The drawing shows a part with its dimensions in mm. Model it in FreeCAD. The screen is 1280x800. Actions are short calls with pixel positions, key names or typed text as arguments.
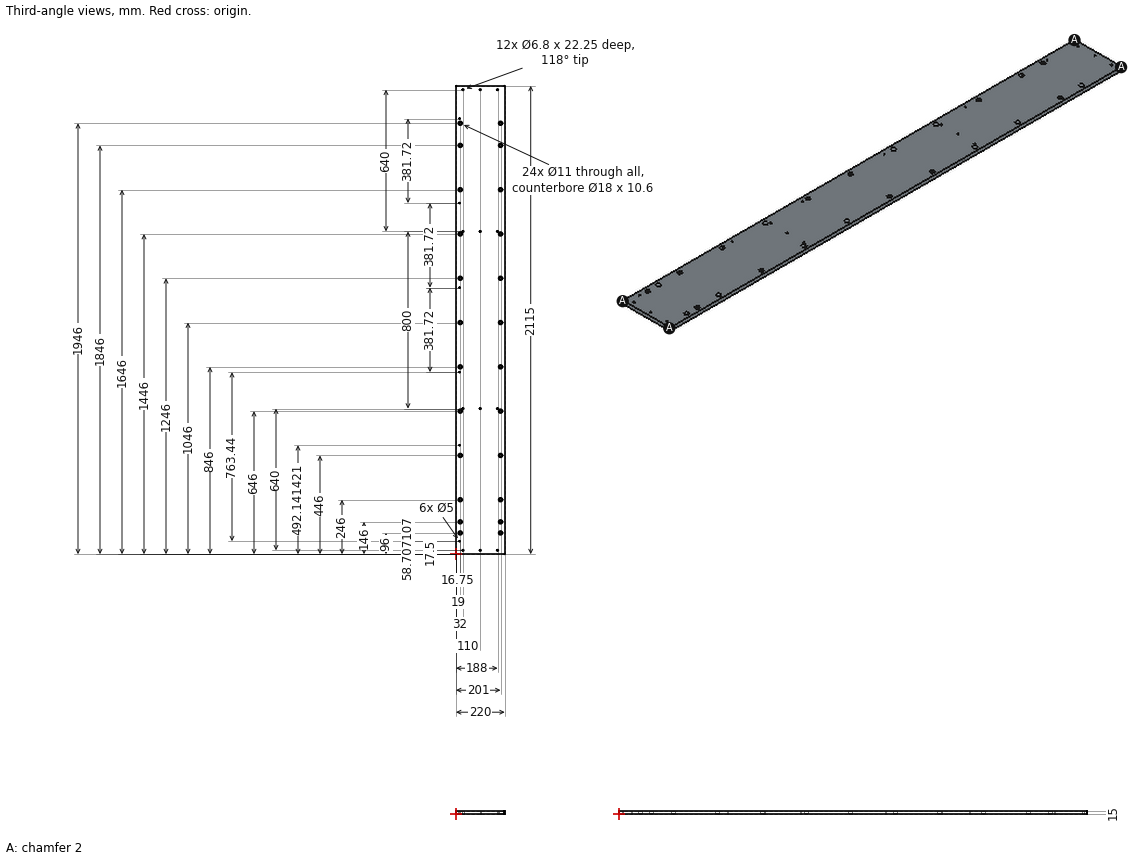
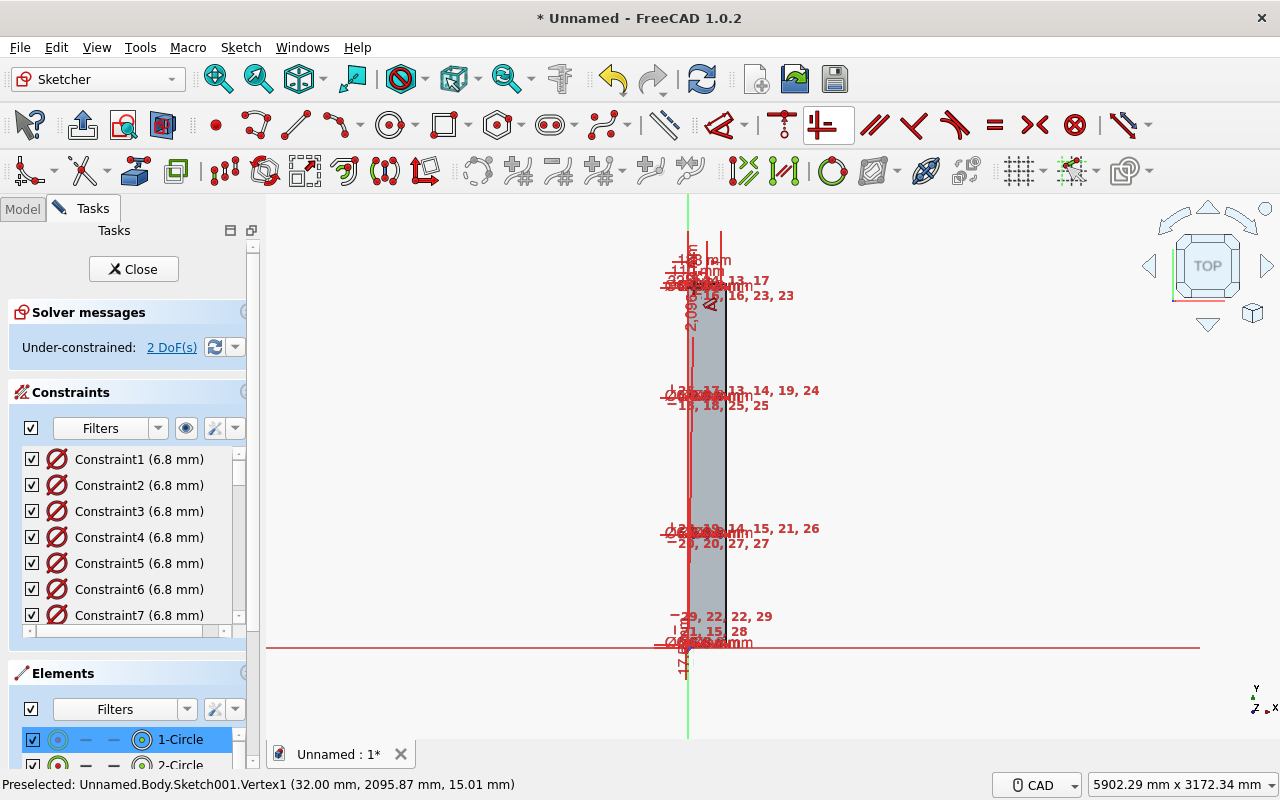
click(694, 398)
click(660, 343)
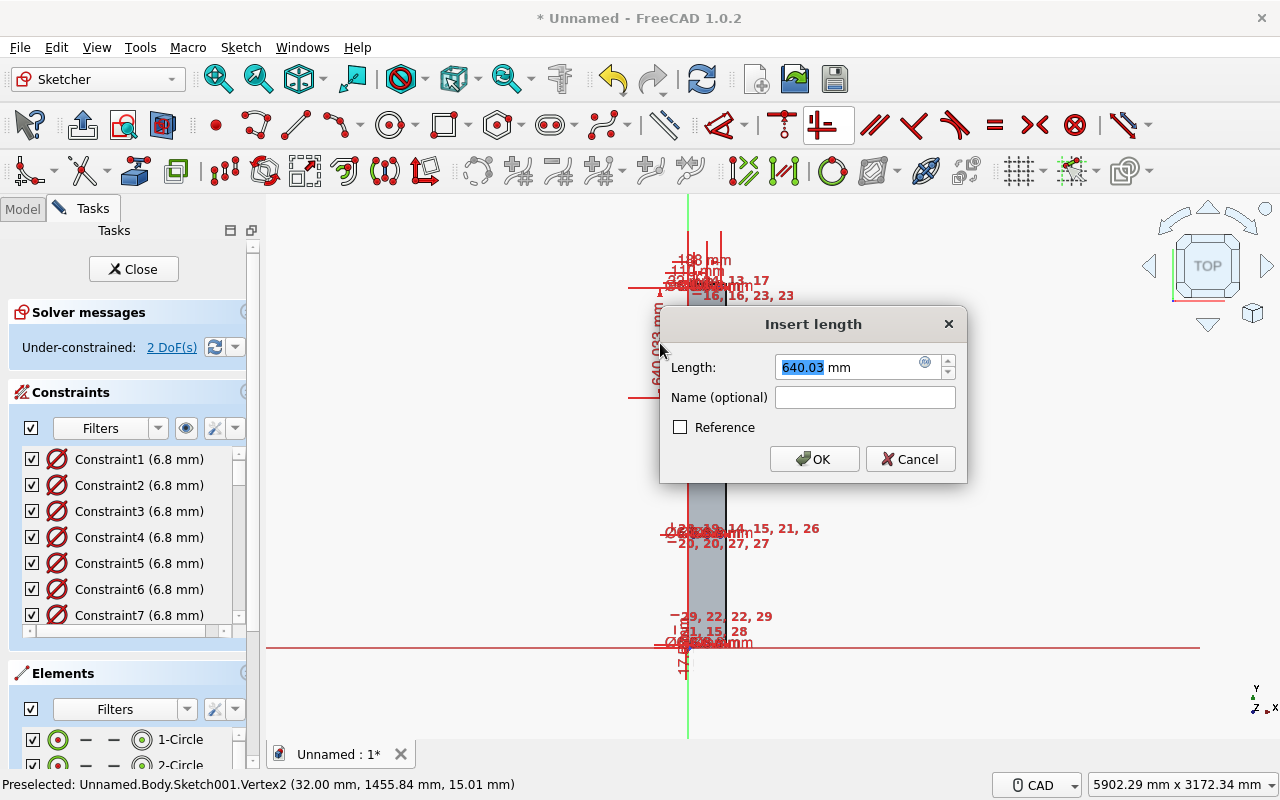
text(640)
key(Return)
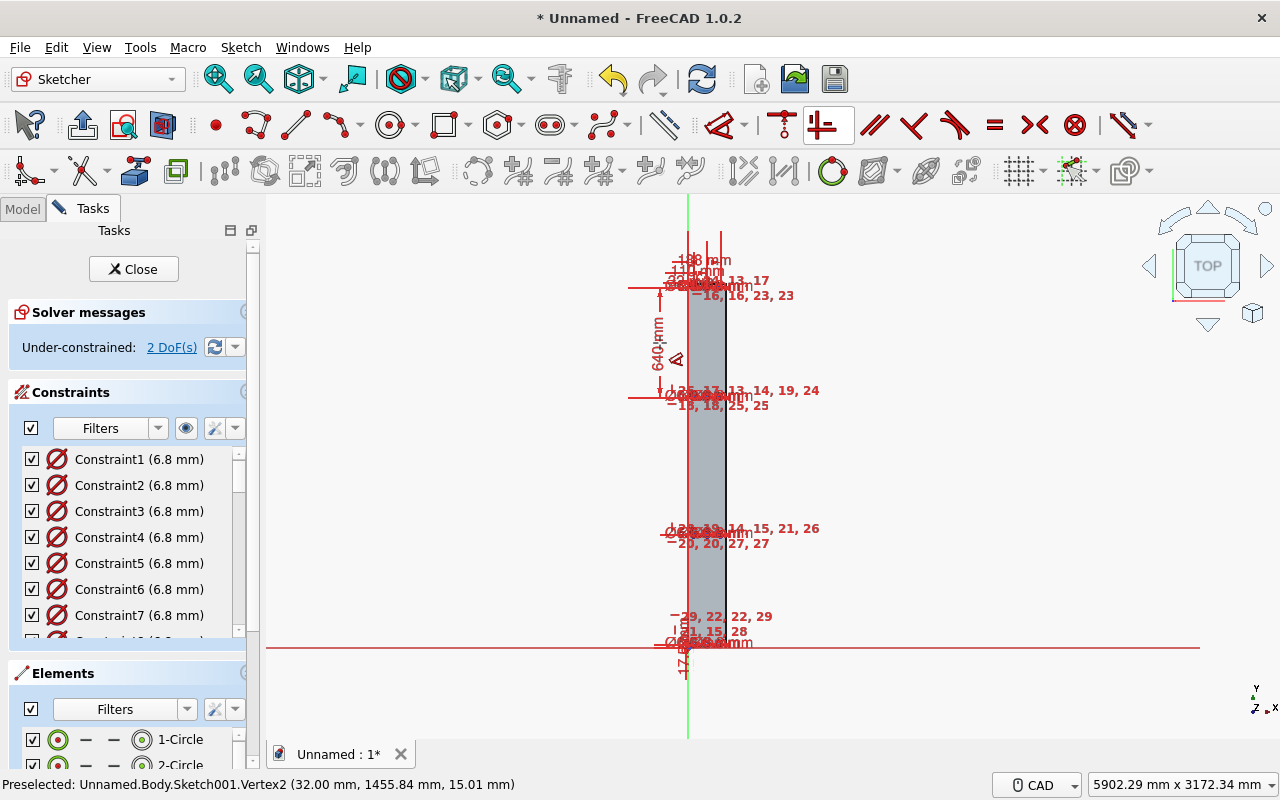
click(694, 398)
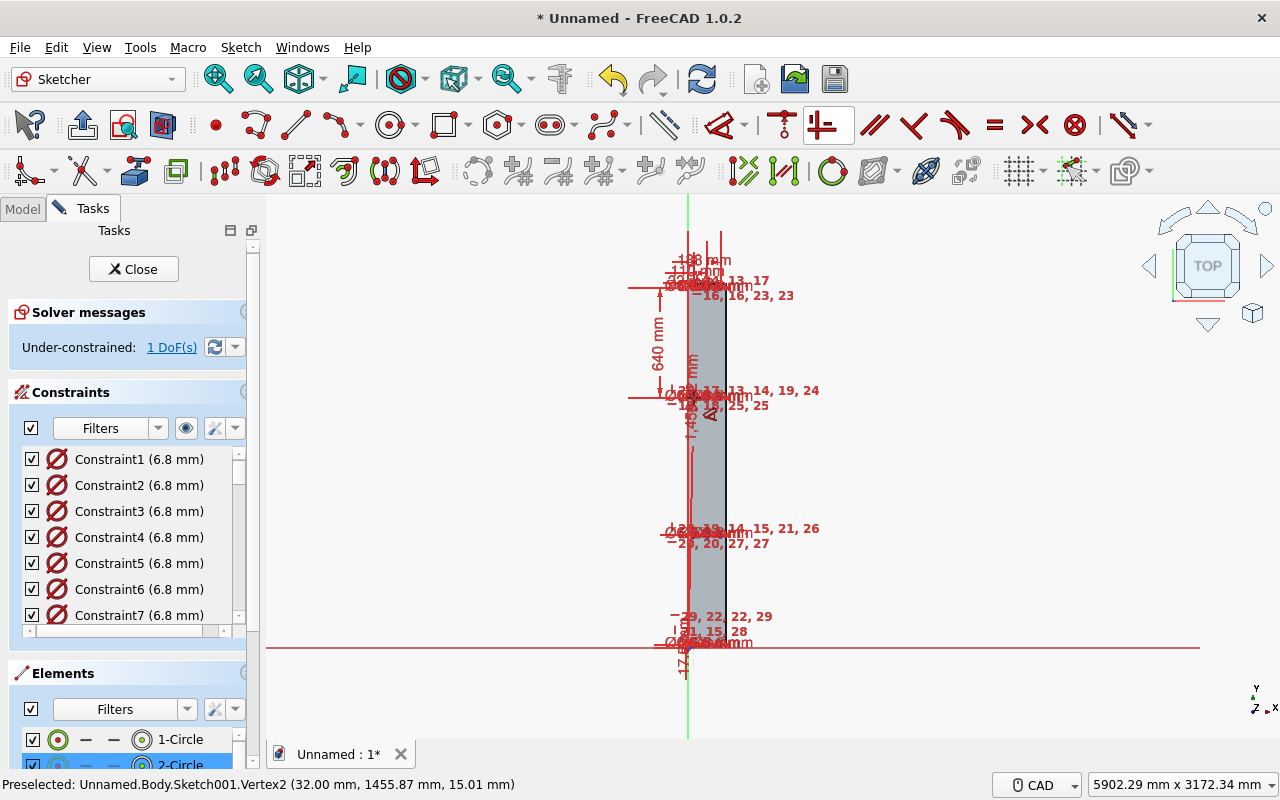
click(694, 535)
click(660, 466)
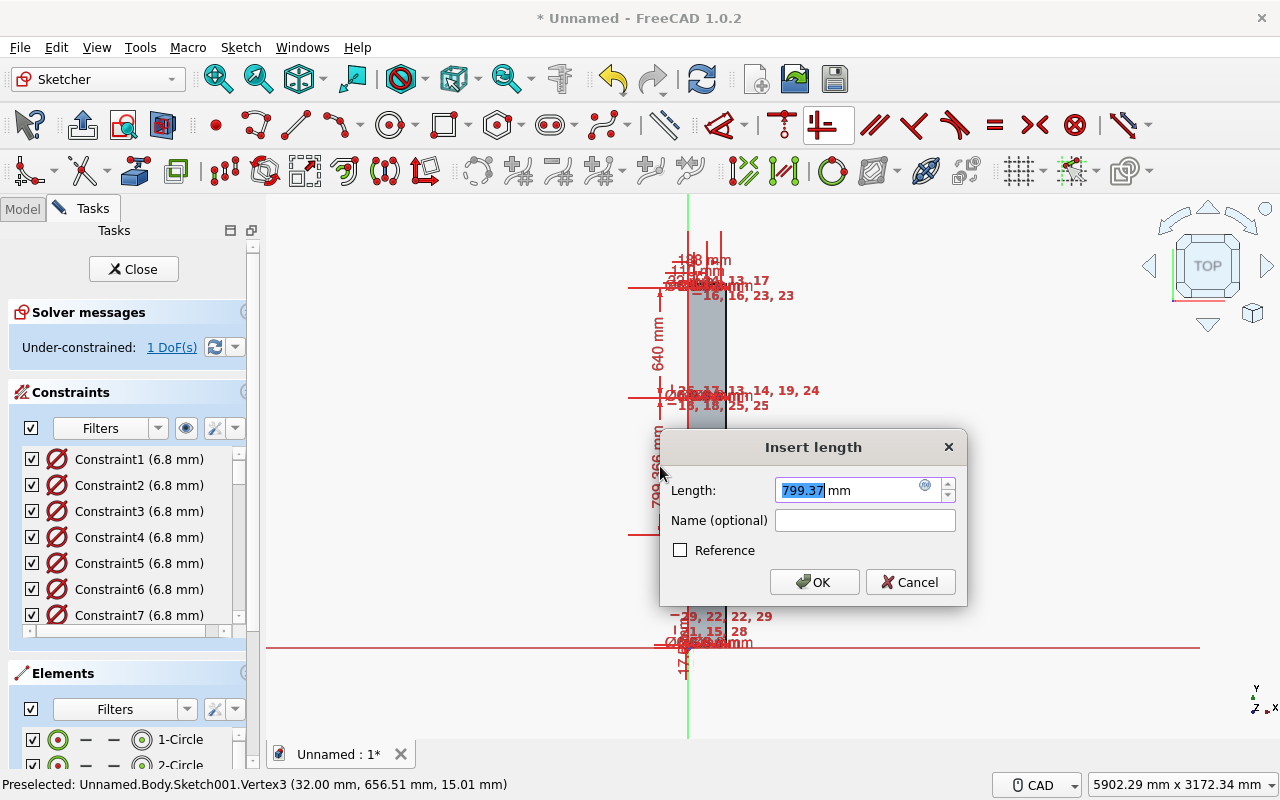
text(800)
key(Return)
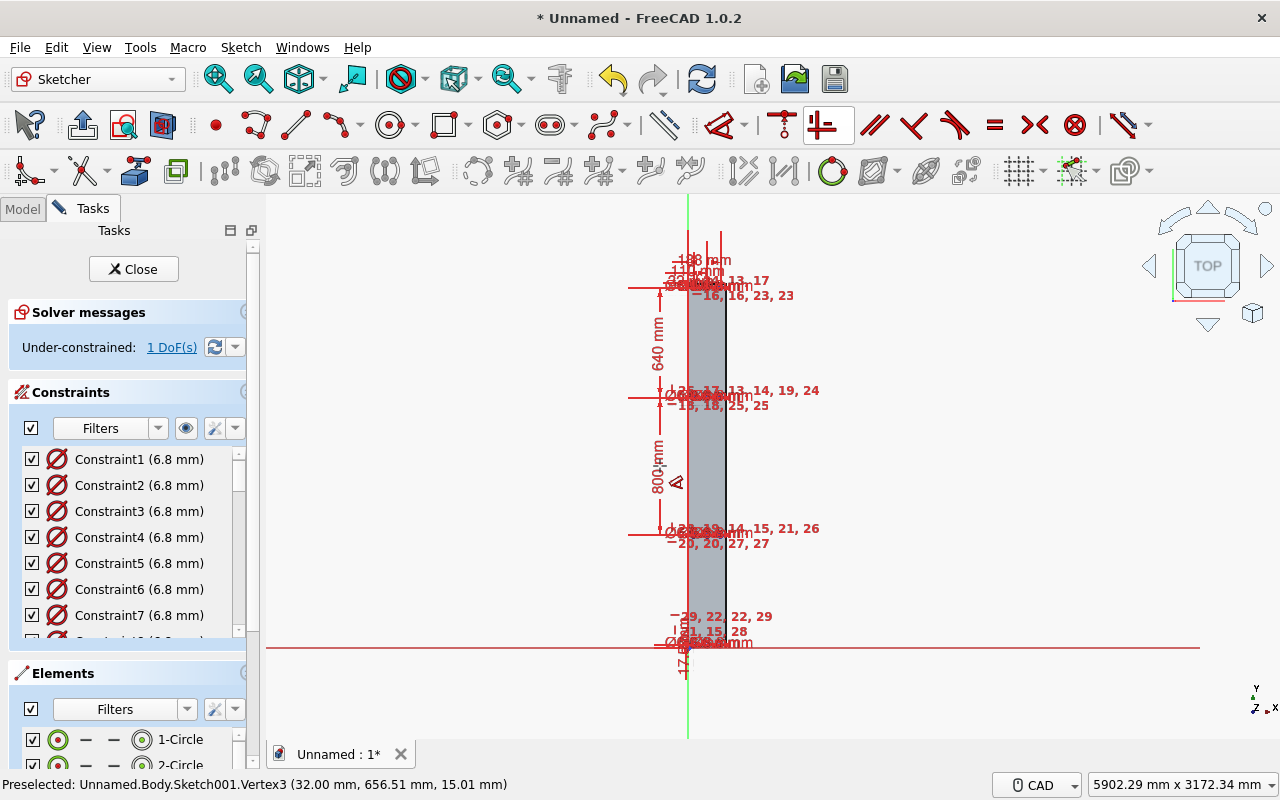
click(694, 535)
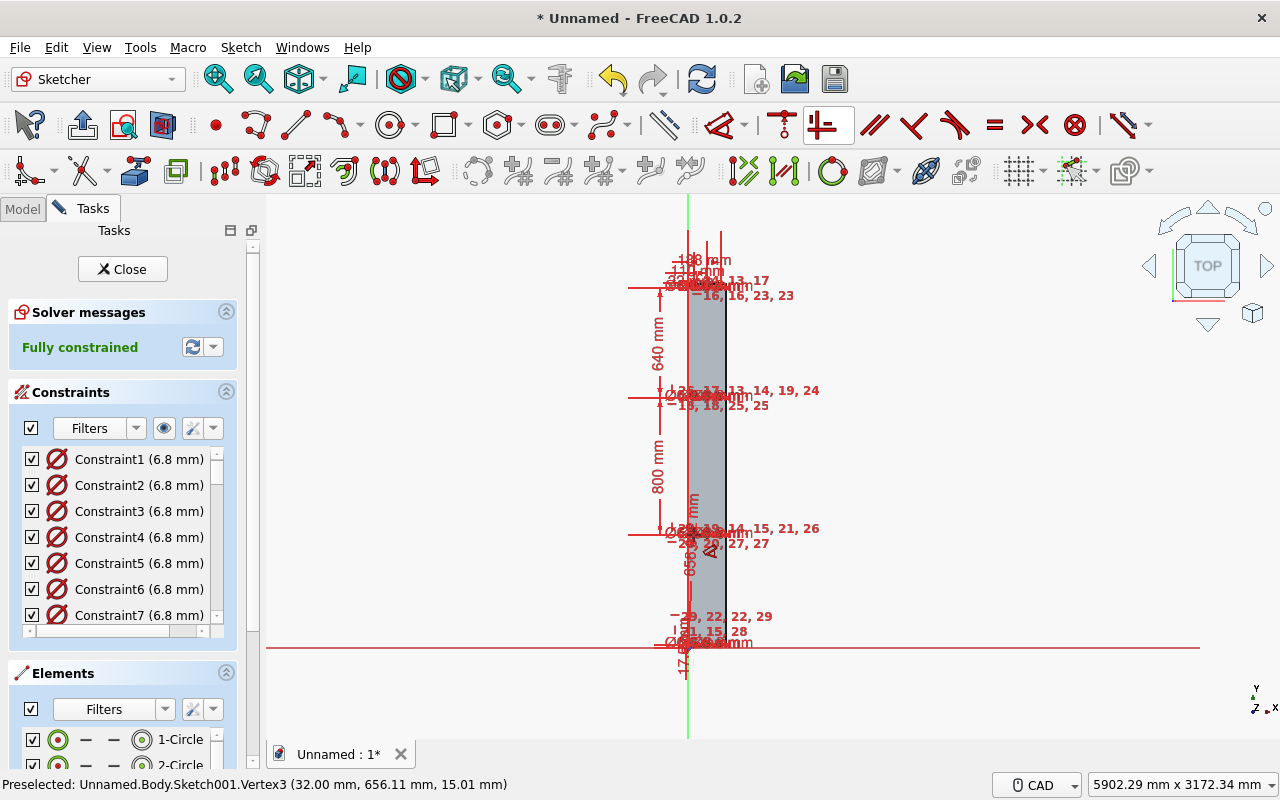
scroll(694, 645, up, 4)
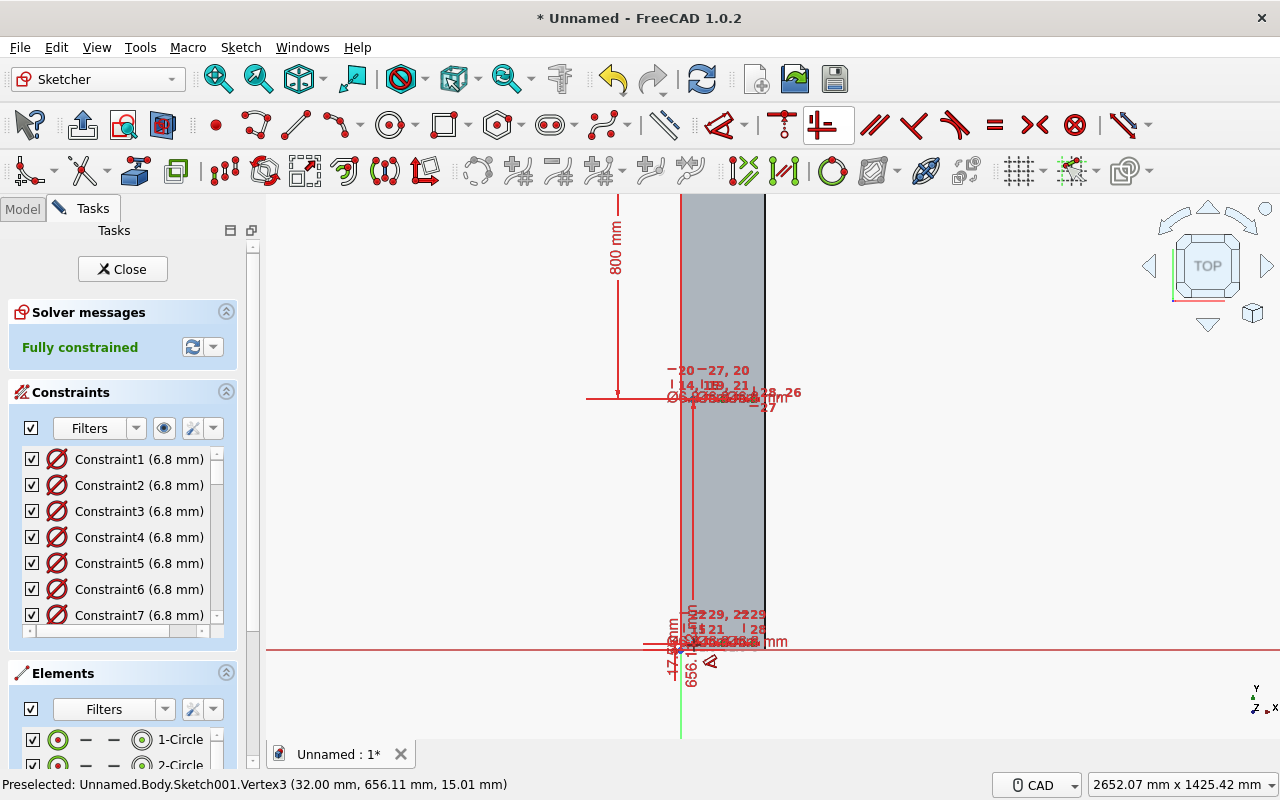
click(693, 644)
click(659, 522)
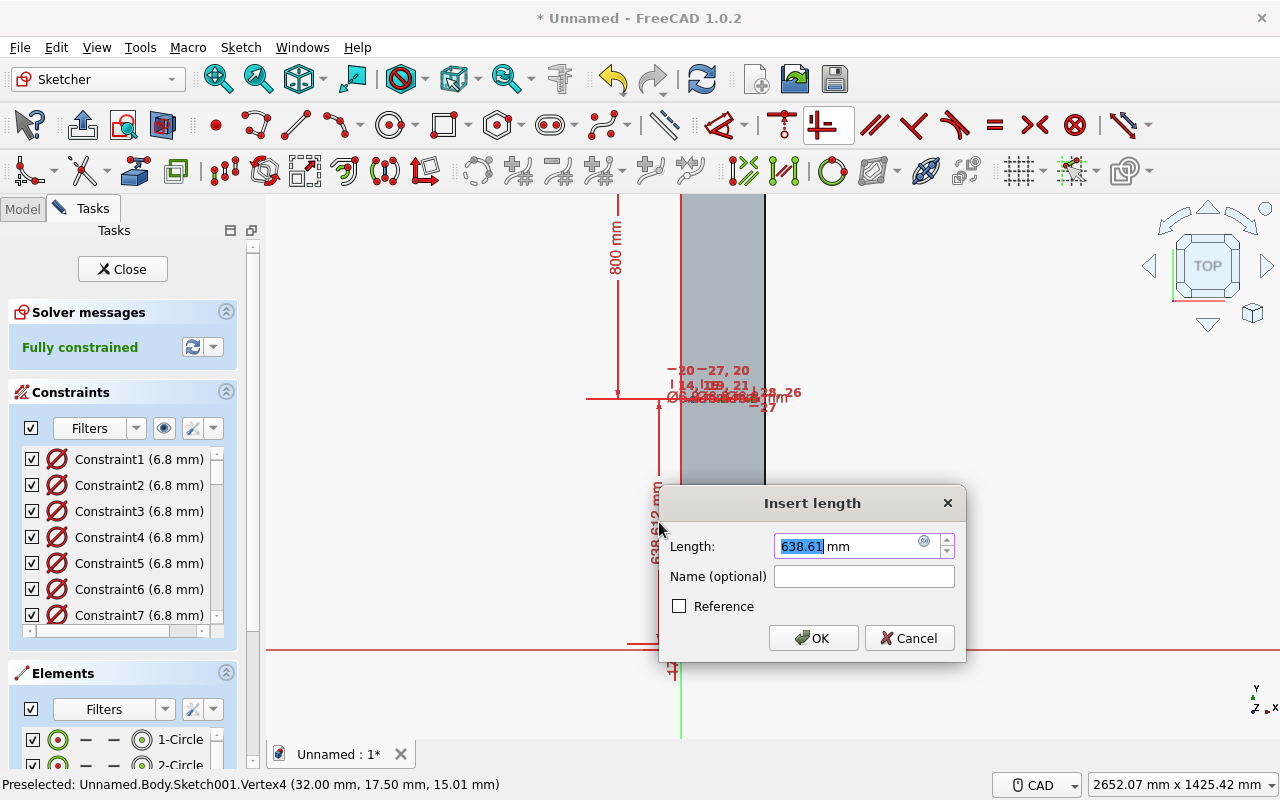
text(640)
key(Return)
key(Escape)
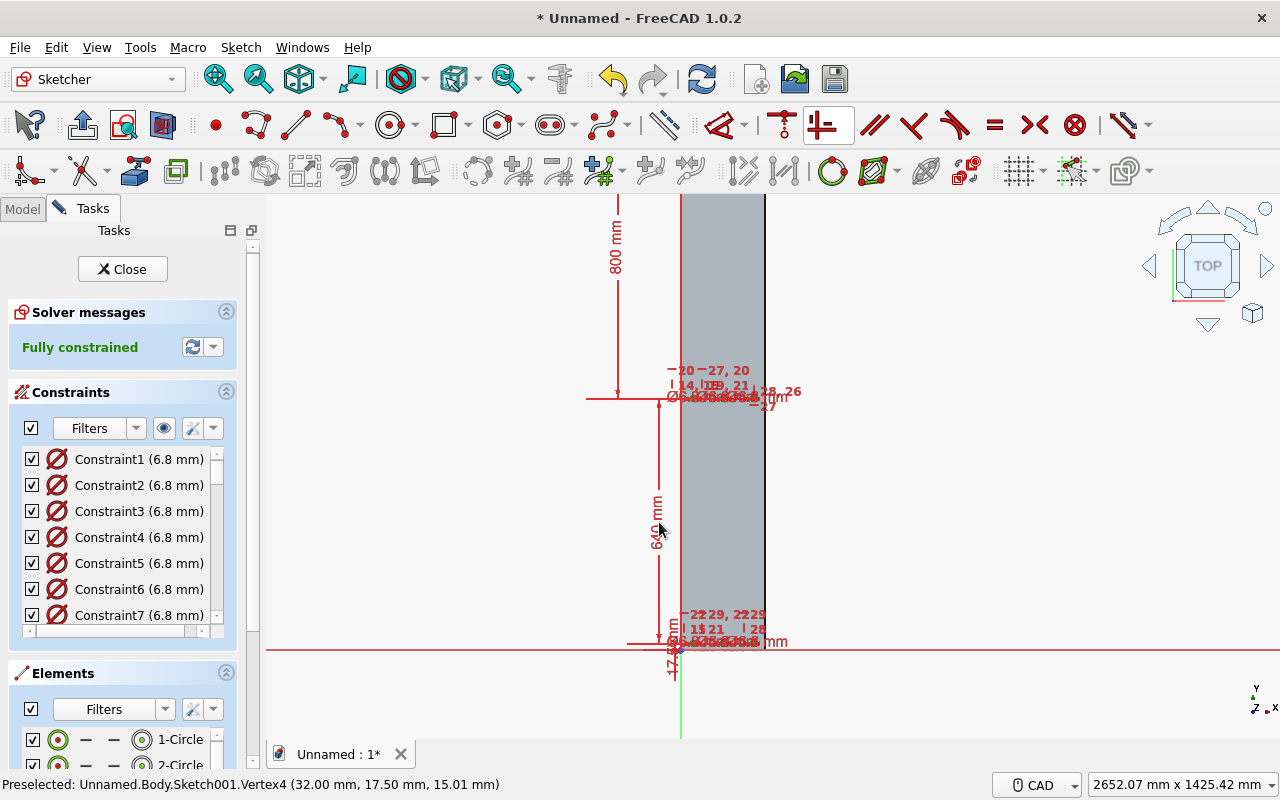
click(123, 269)